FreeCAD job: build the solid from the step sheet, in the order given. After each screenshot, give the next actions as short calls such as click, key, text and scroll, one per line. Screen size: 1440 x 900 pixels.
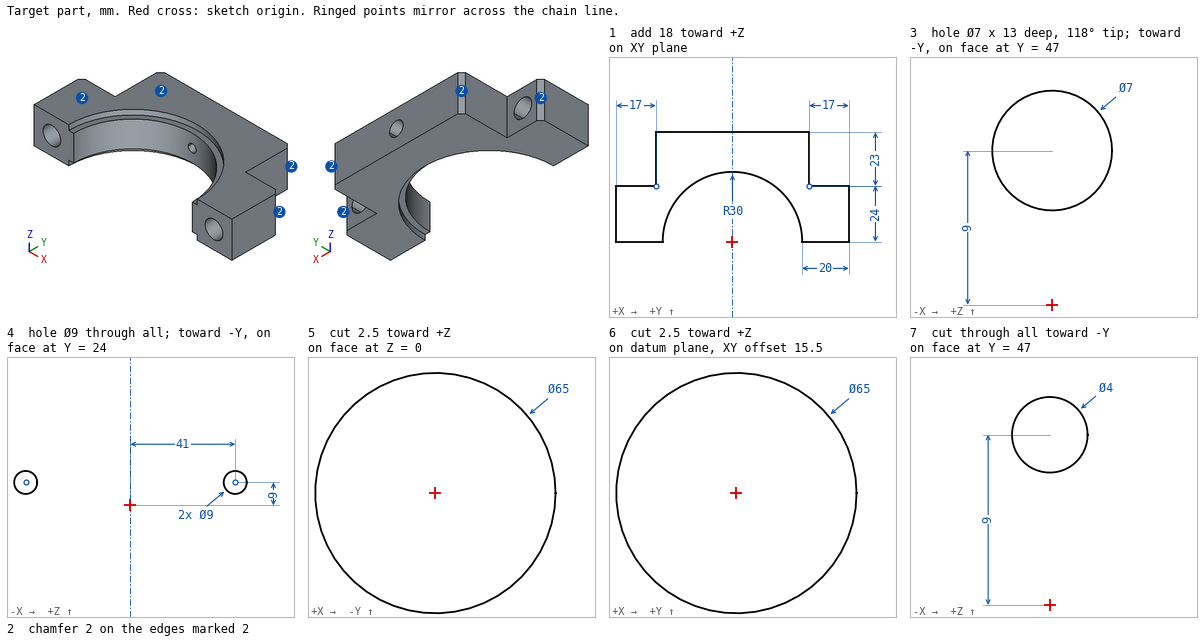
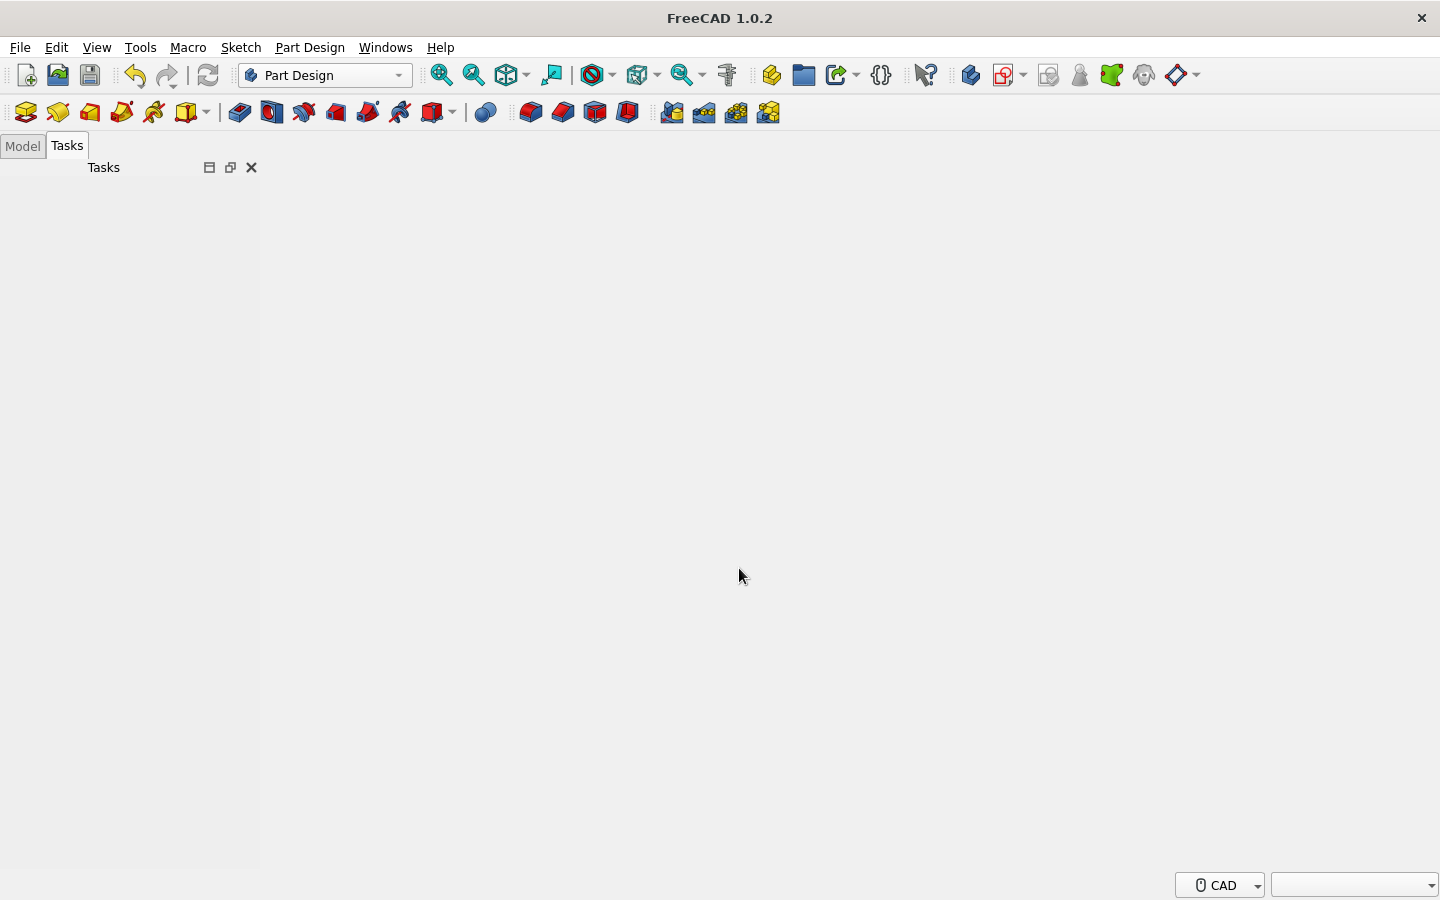
key(ctrl+n)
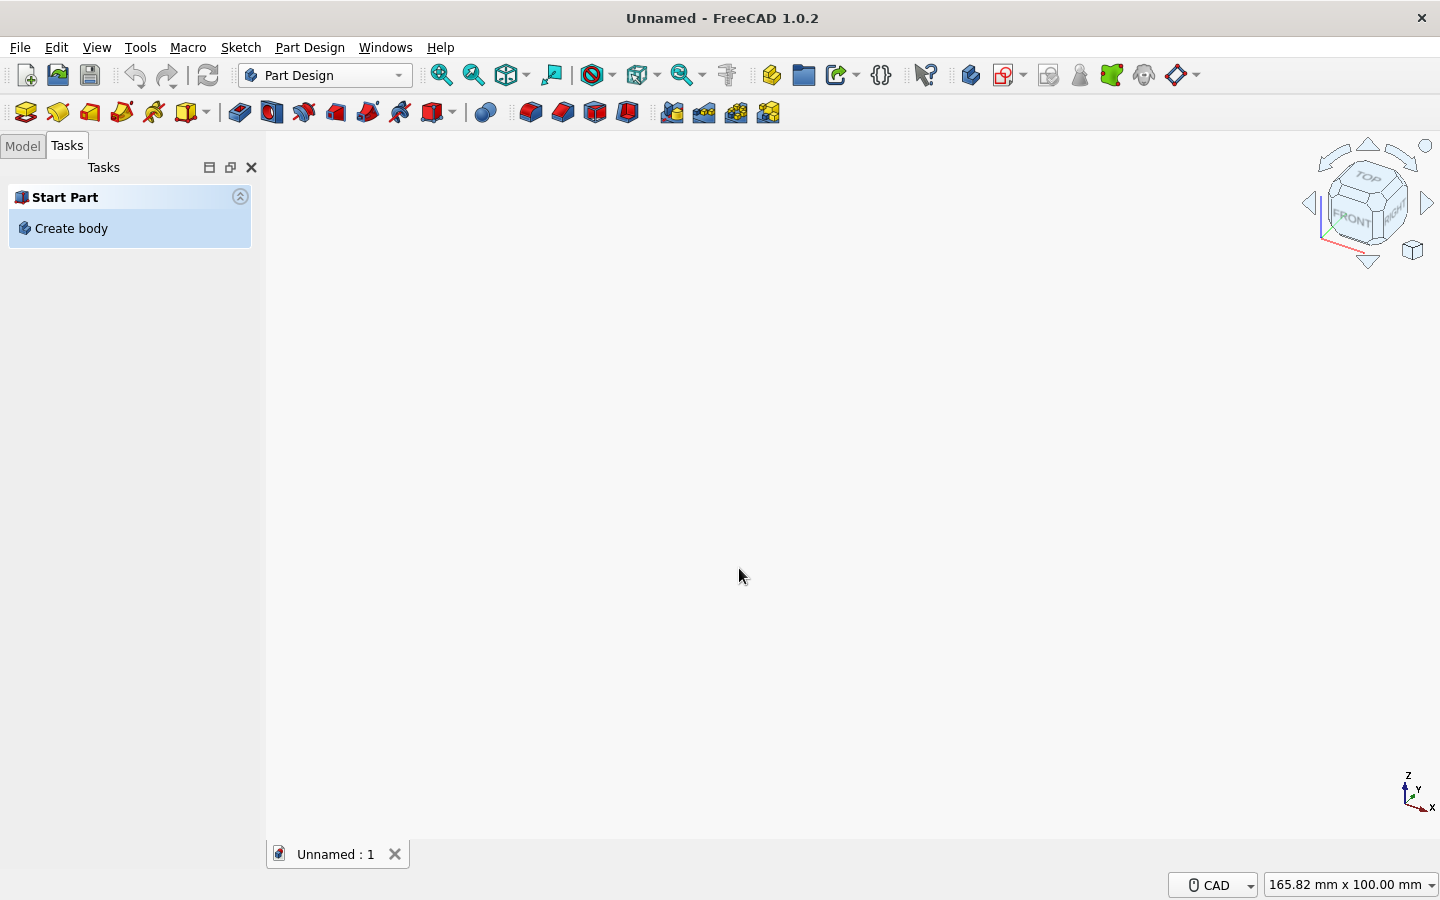
click(1004, 76)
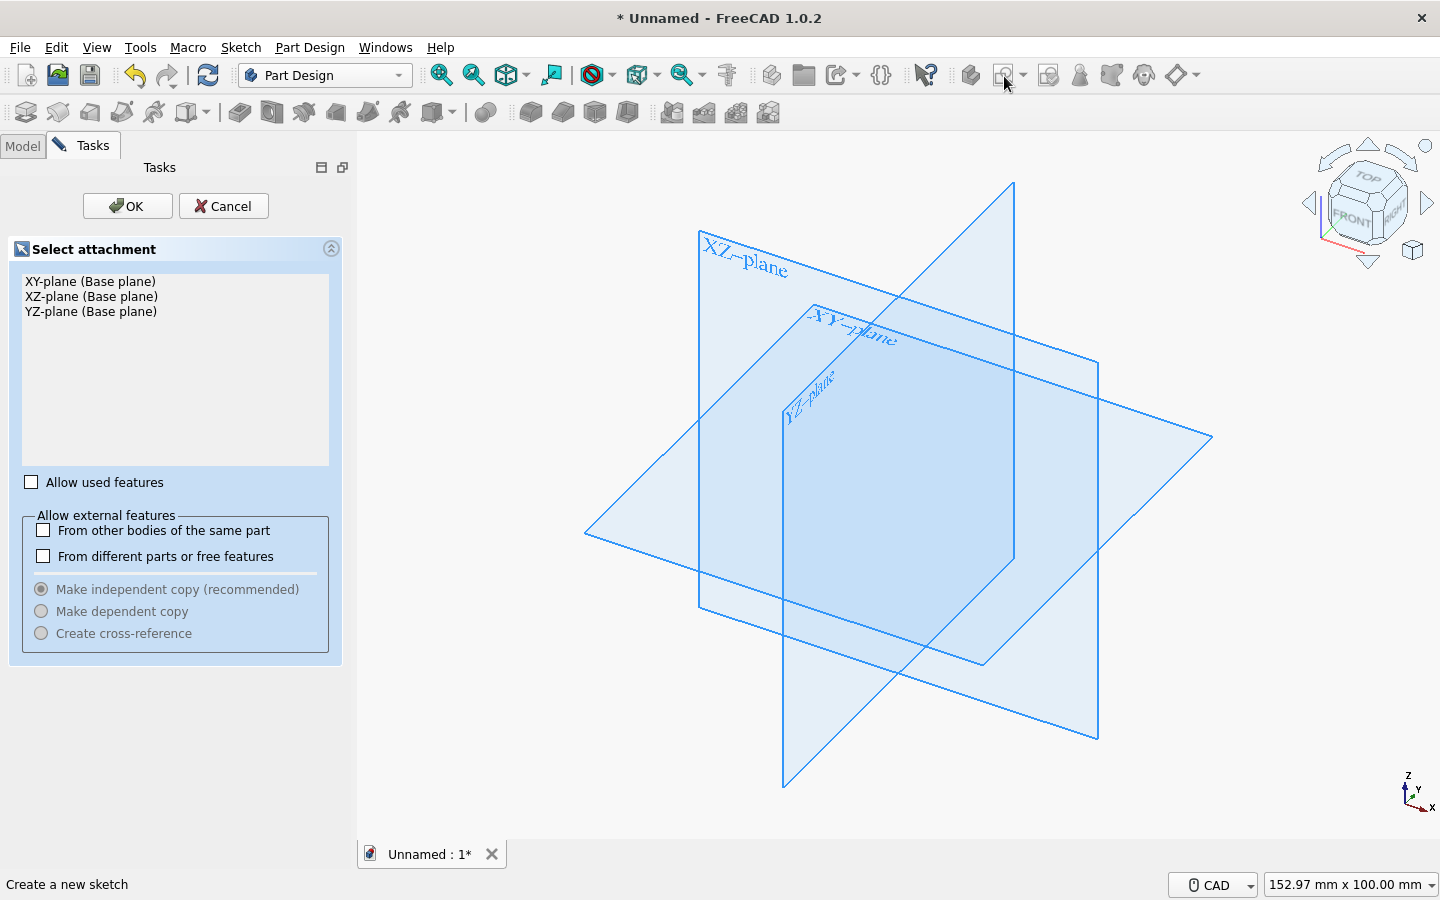
click(82, 282)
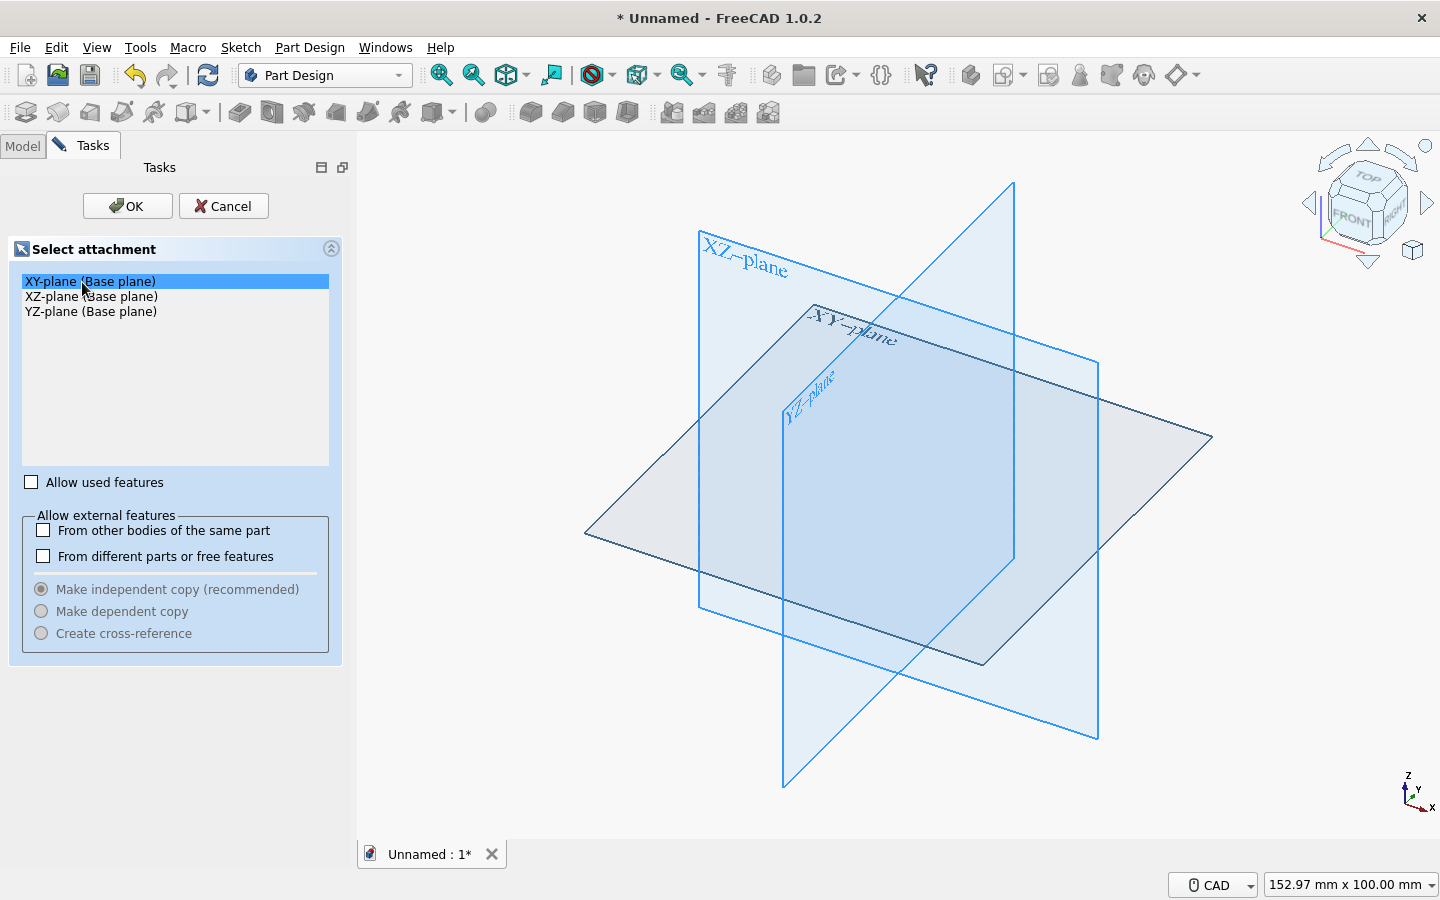
click(128, 206)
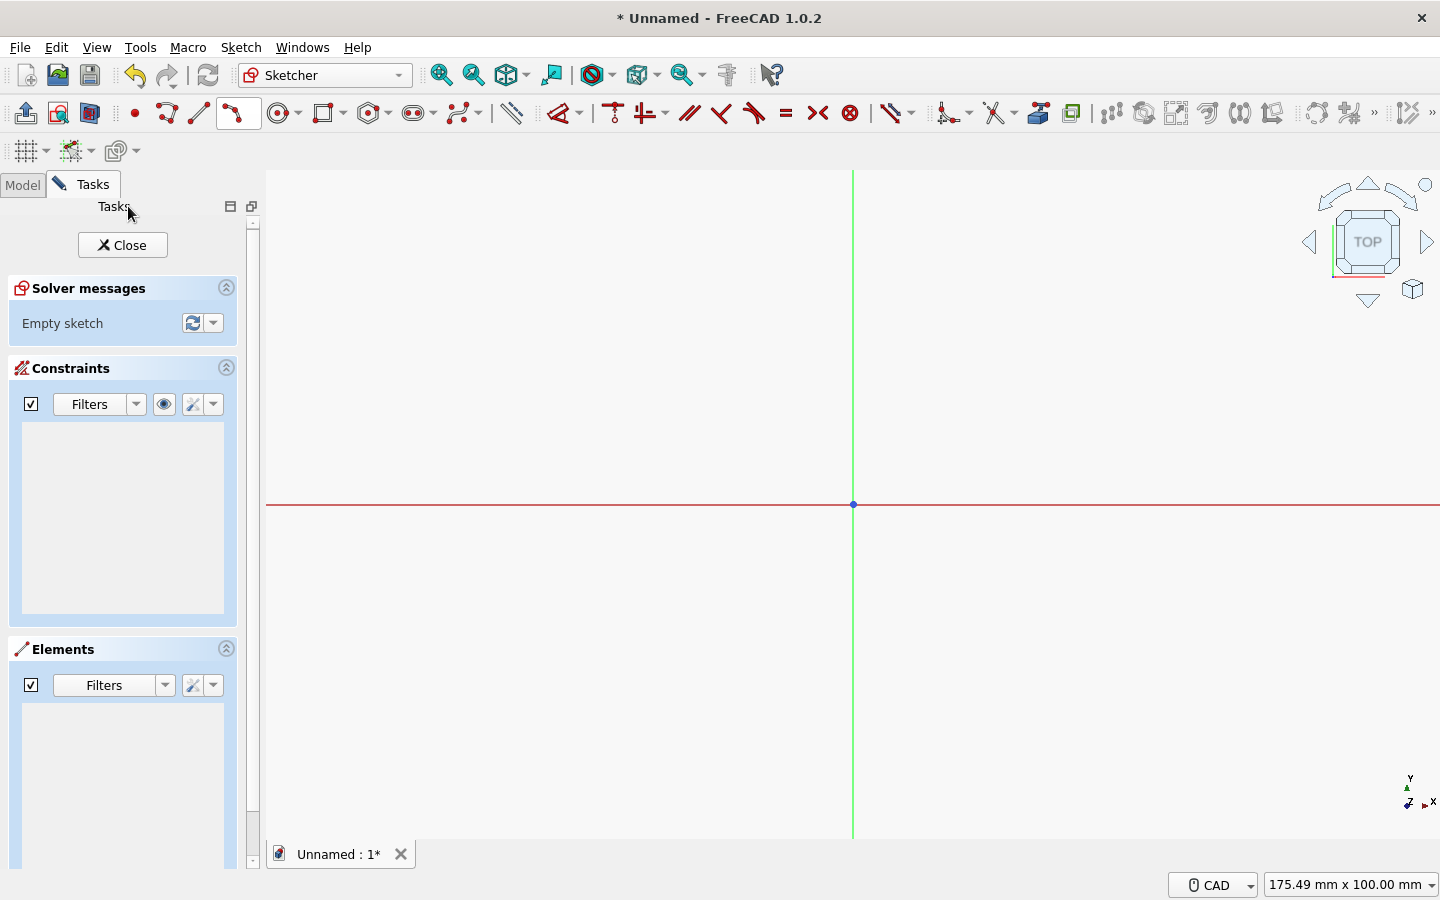
scroll(475, 811, down, 1)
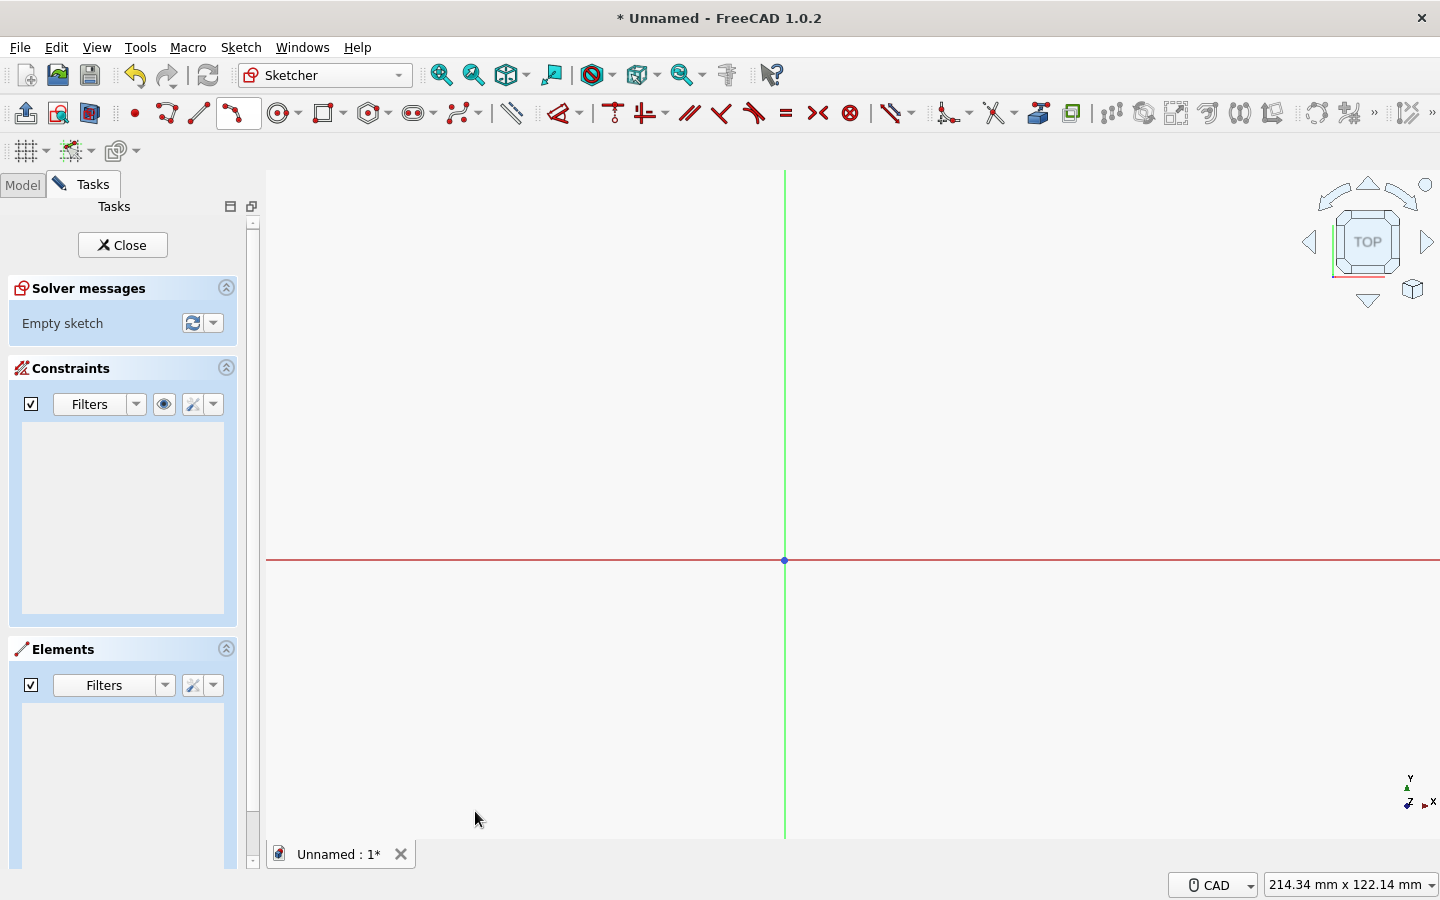
click(168, 114)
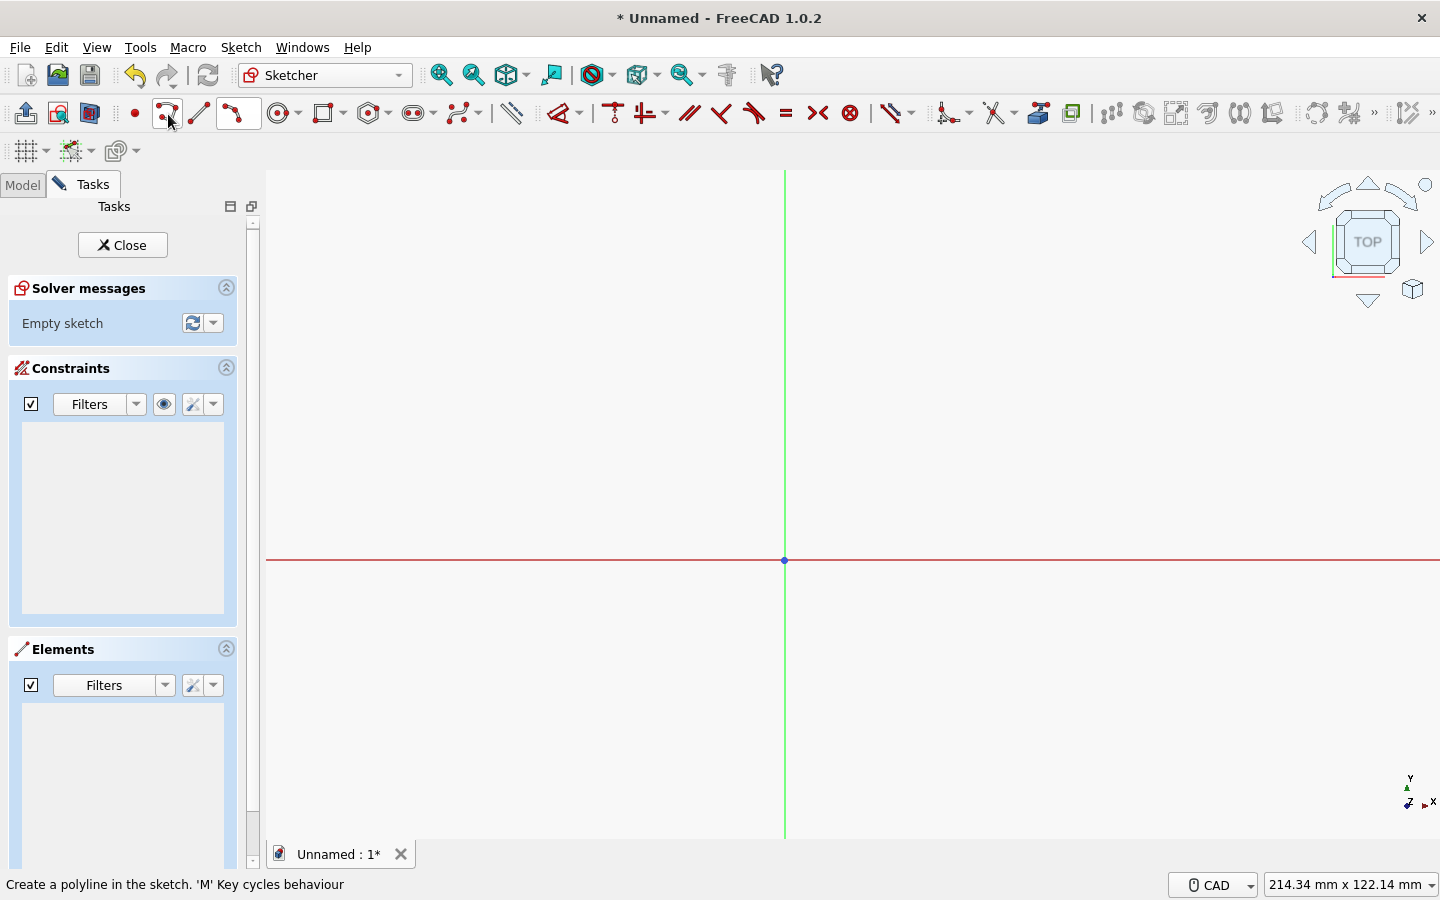
click(949, 560)
click(1058, 551)
click(1058, 429)
click(965, 429)
click(965, 303)
click(604, 303)
click(604, 429)
click(511, 429)
click(511, 560)
click(620, 551)
right_click(620, 551)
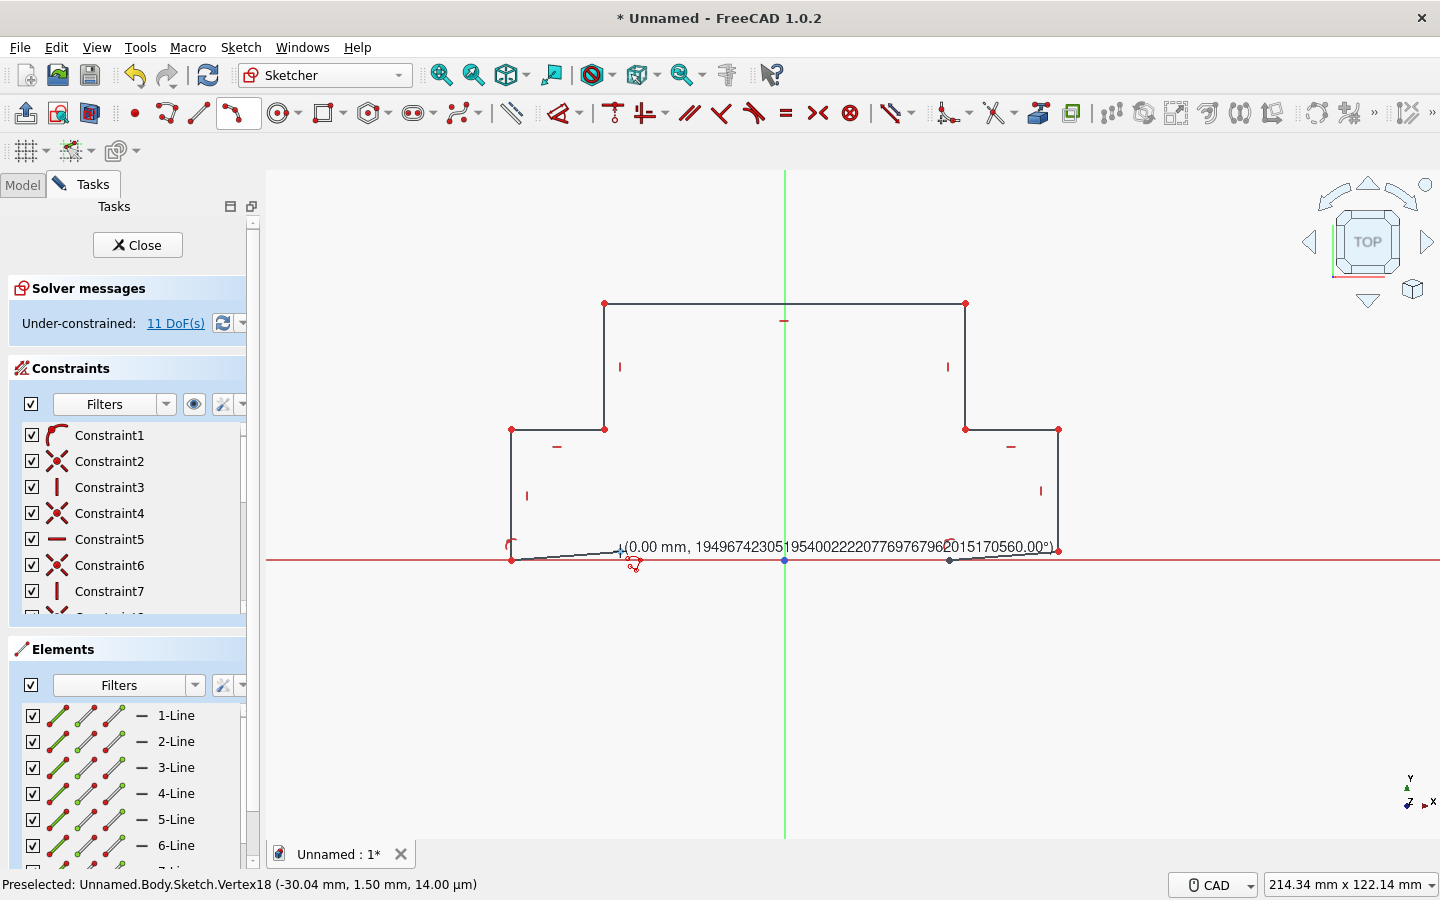
click(232, 114)